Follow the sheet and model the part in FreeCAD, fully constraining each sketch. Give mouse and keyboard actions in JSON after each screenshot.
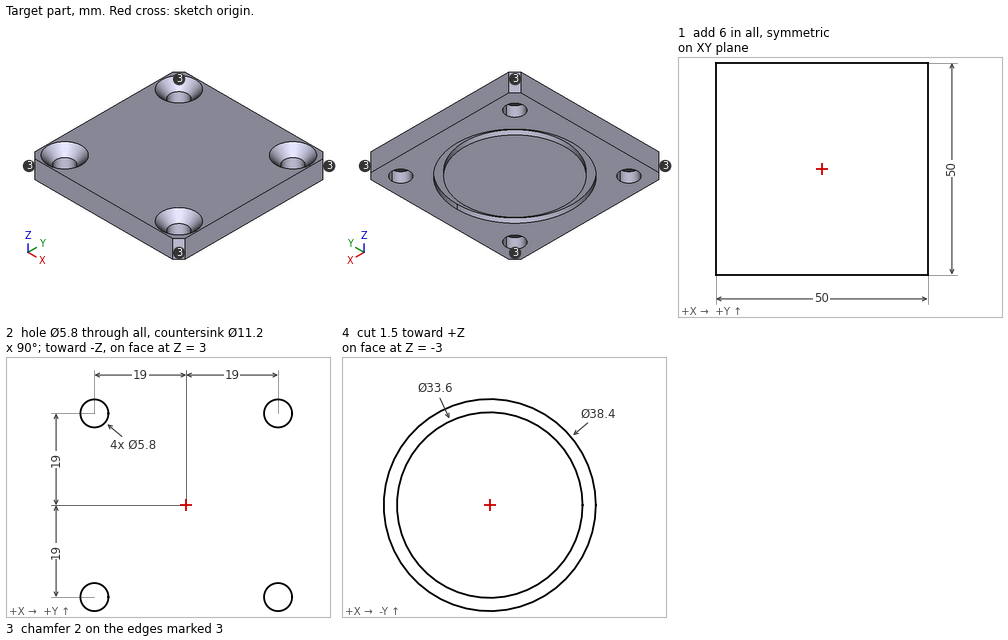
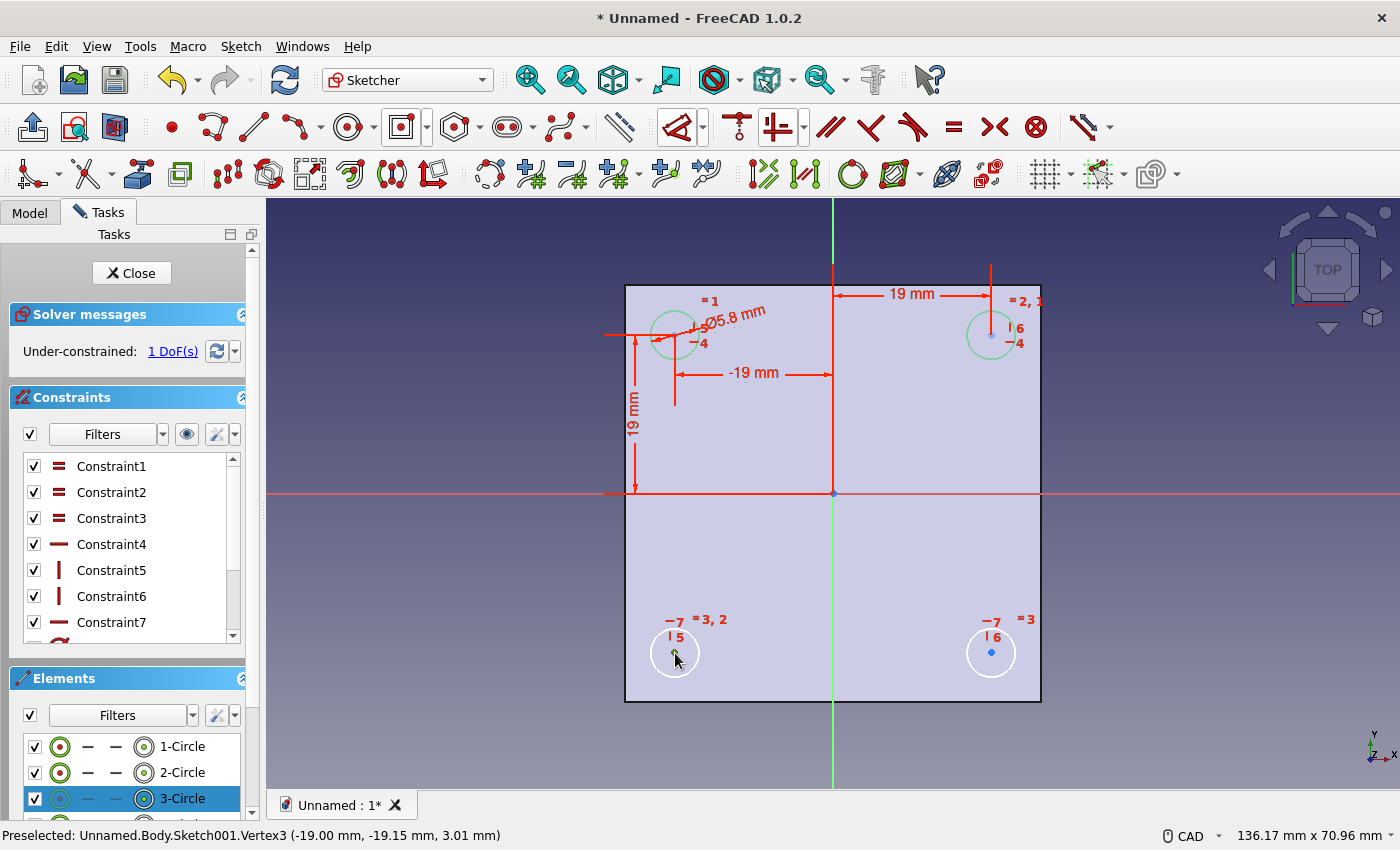
{"action": "key", "text": "i"}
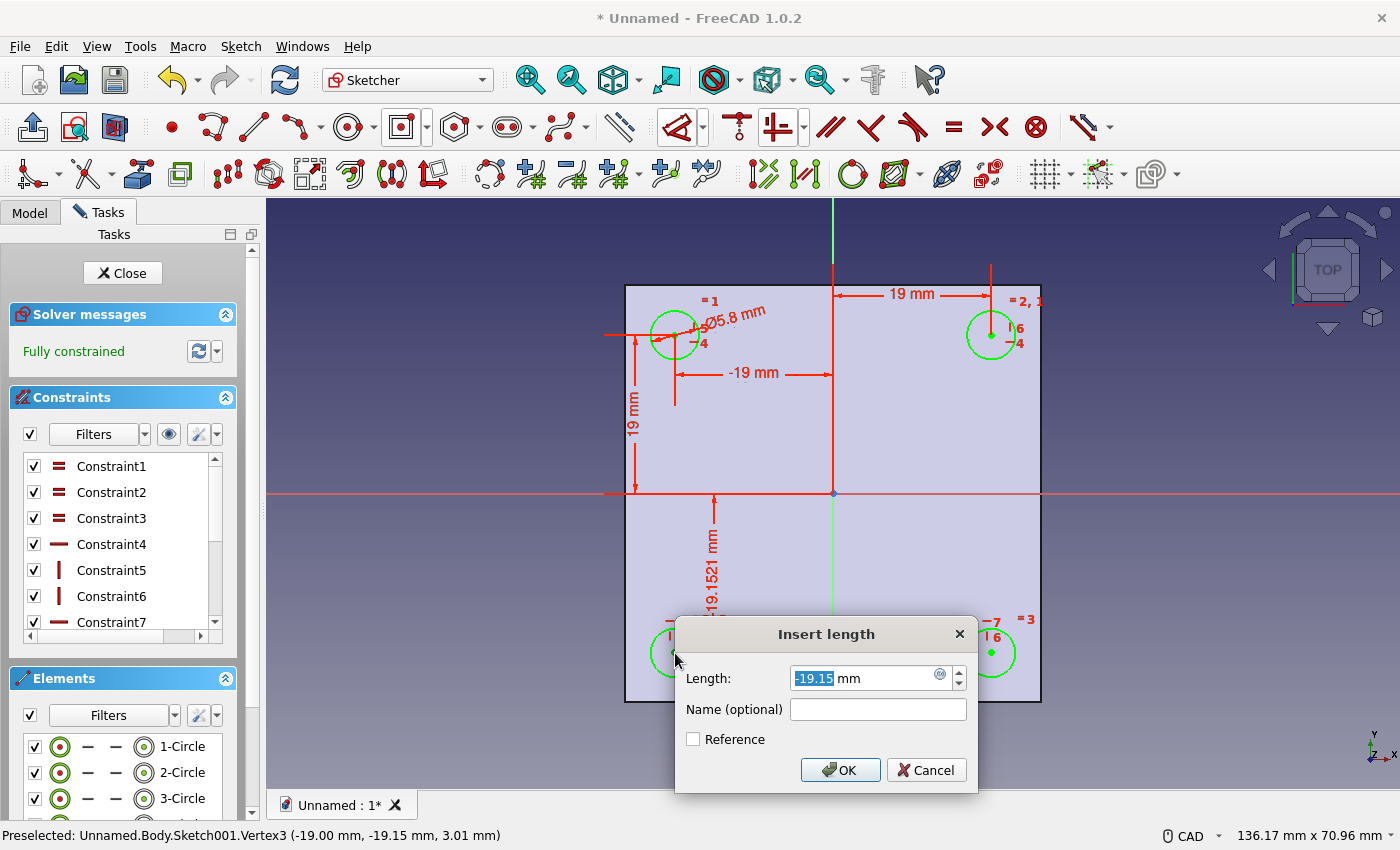
{"action": "type", "text": "-19"}
{"action": "key", "text": "Return"}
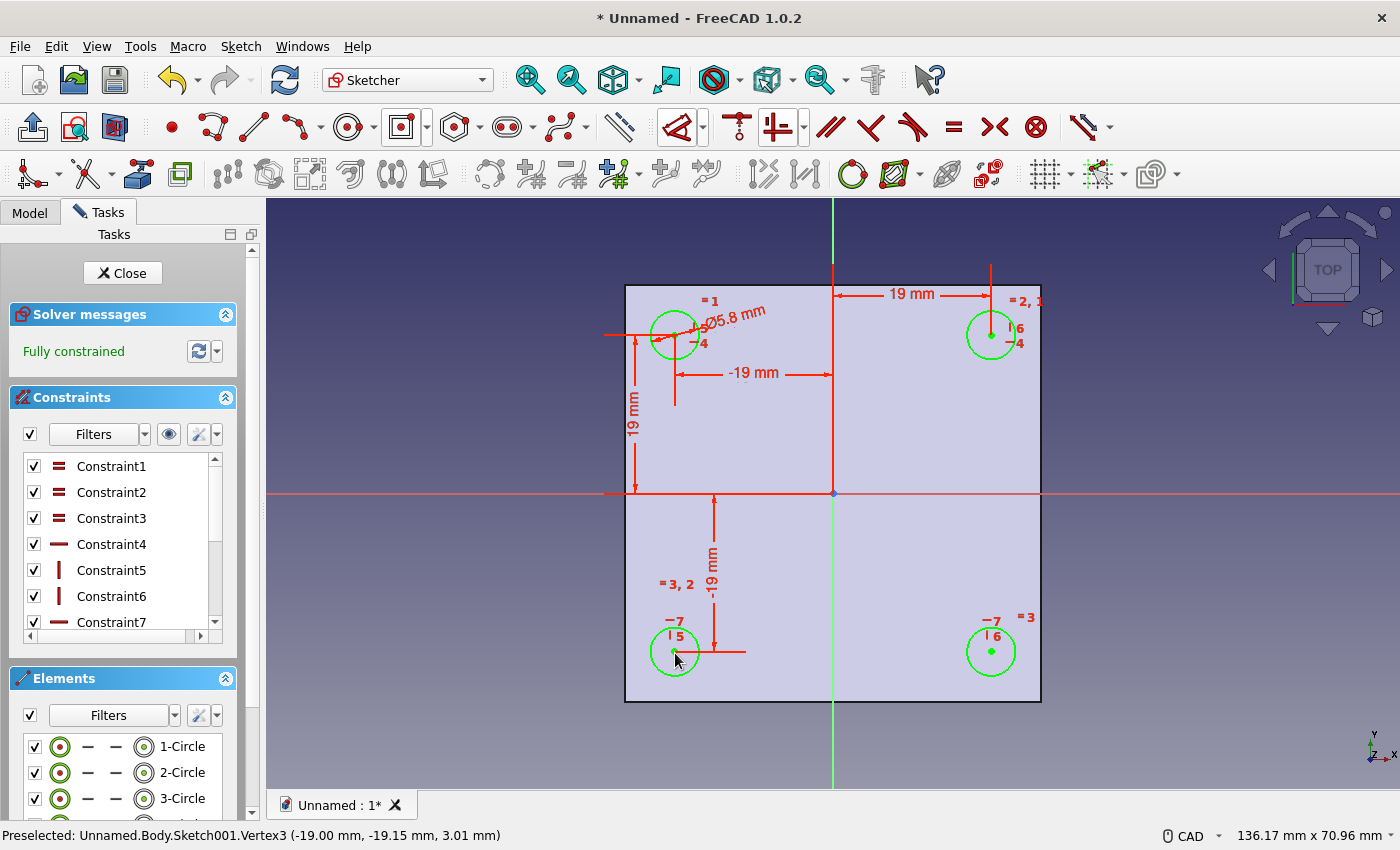
{"action": "left_click", "coordinate": [123, 273]}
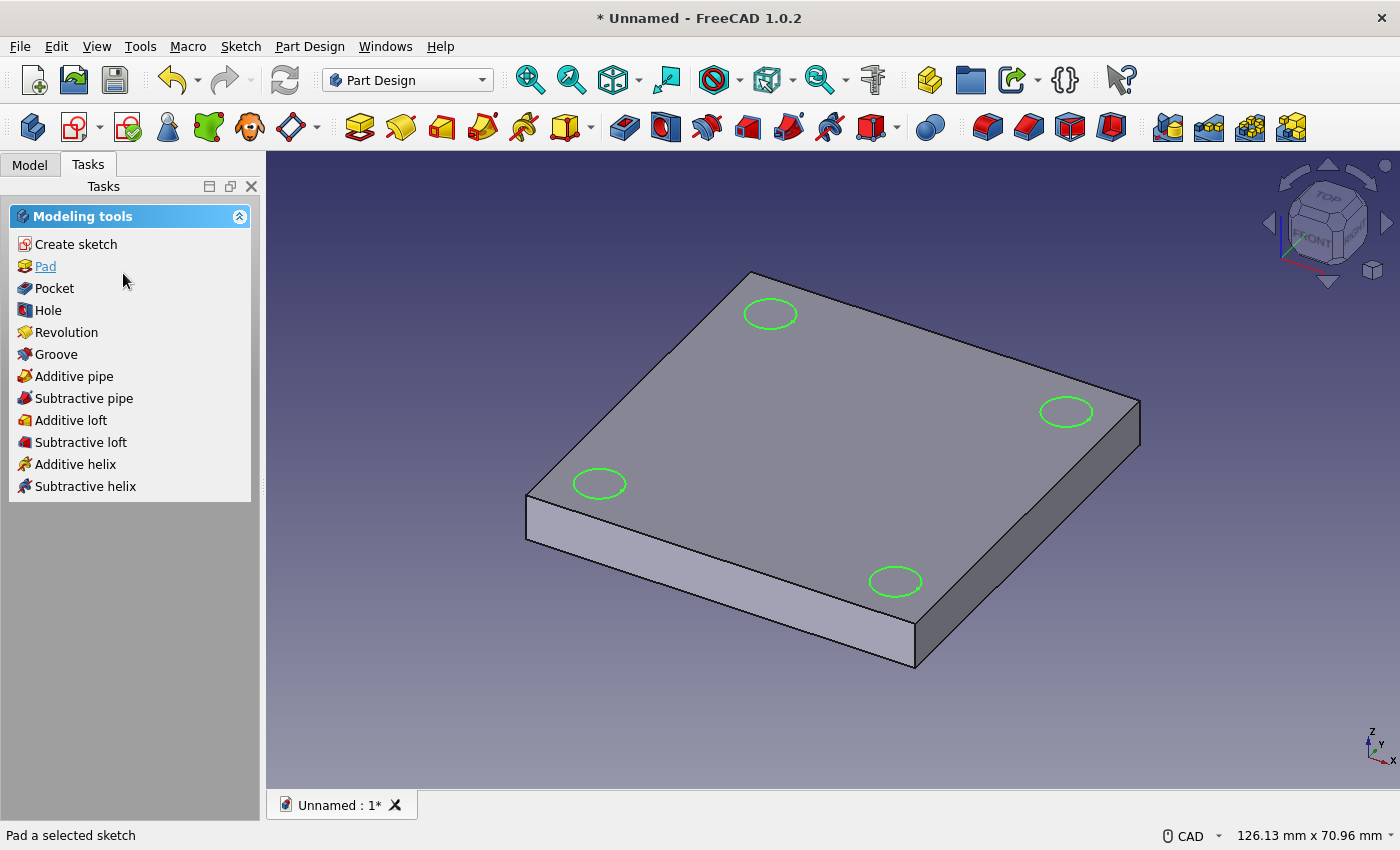
{"action": "left_click", "coordinate": [666, 128]}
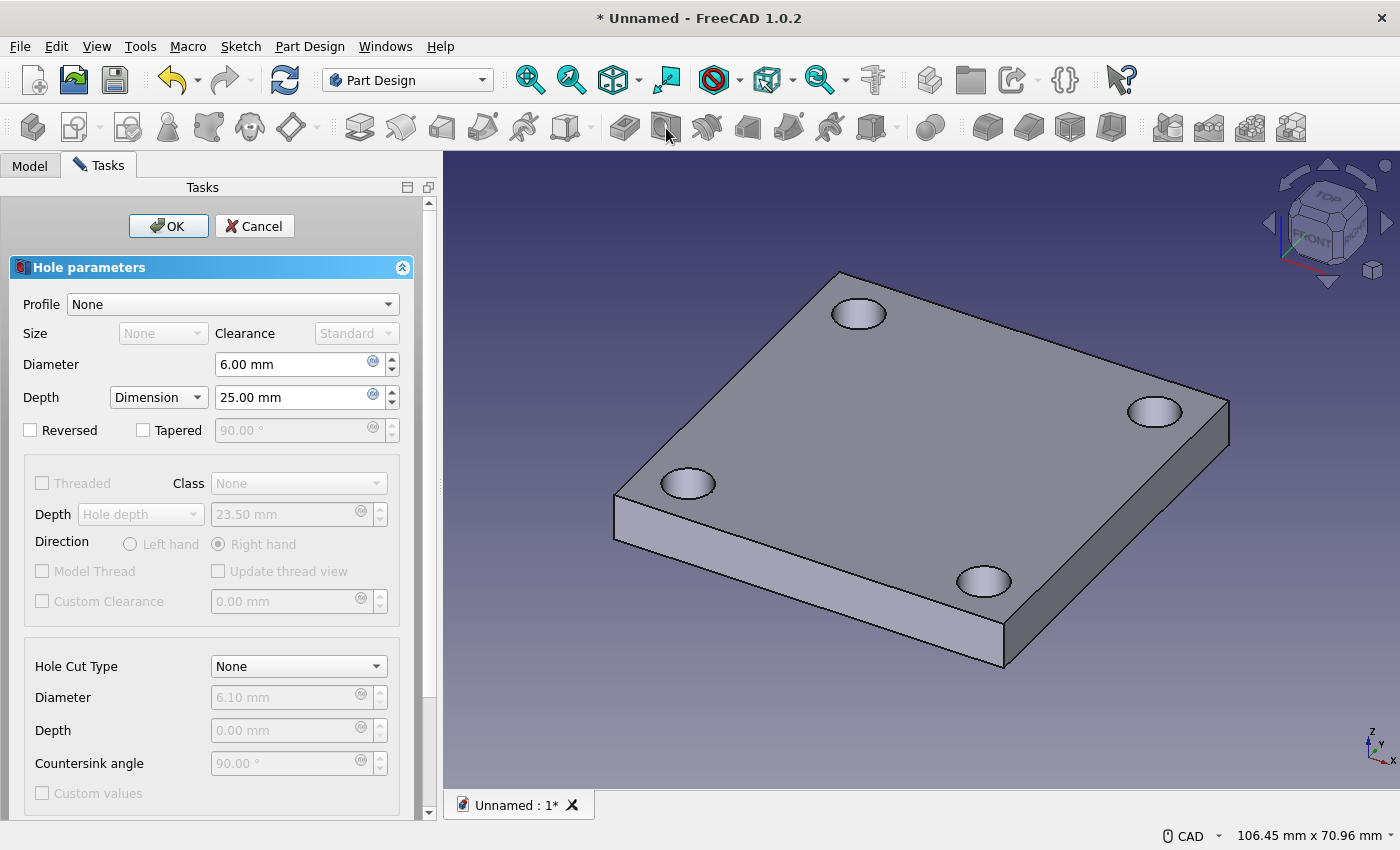
{"action": "triple_click", "coordinate": [300, 364]}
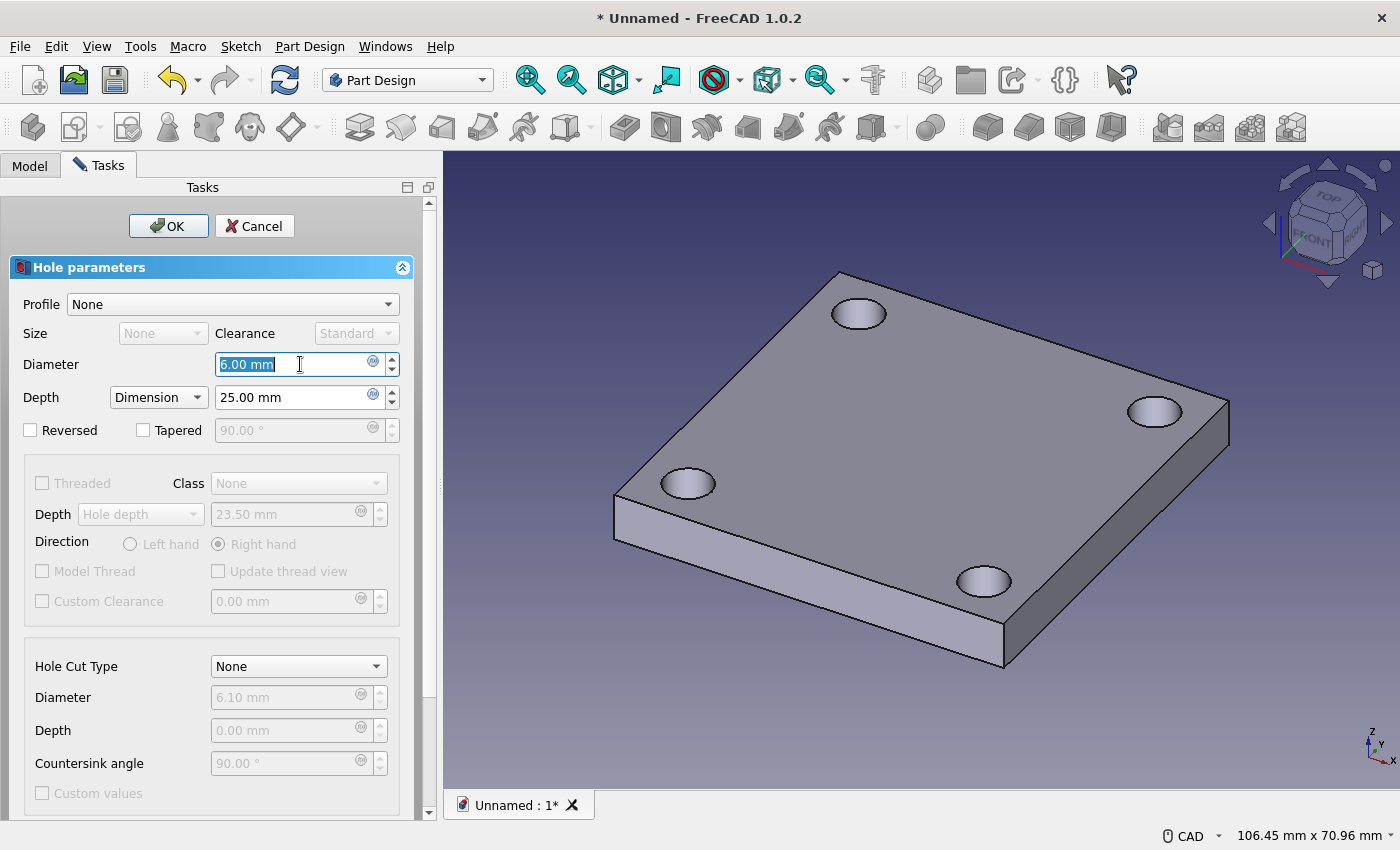
{"action": "type", "text": "5.8"}
{"action": "key", "text": "Tab"}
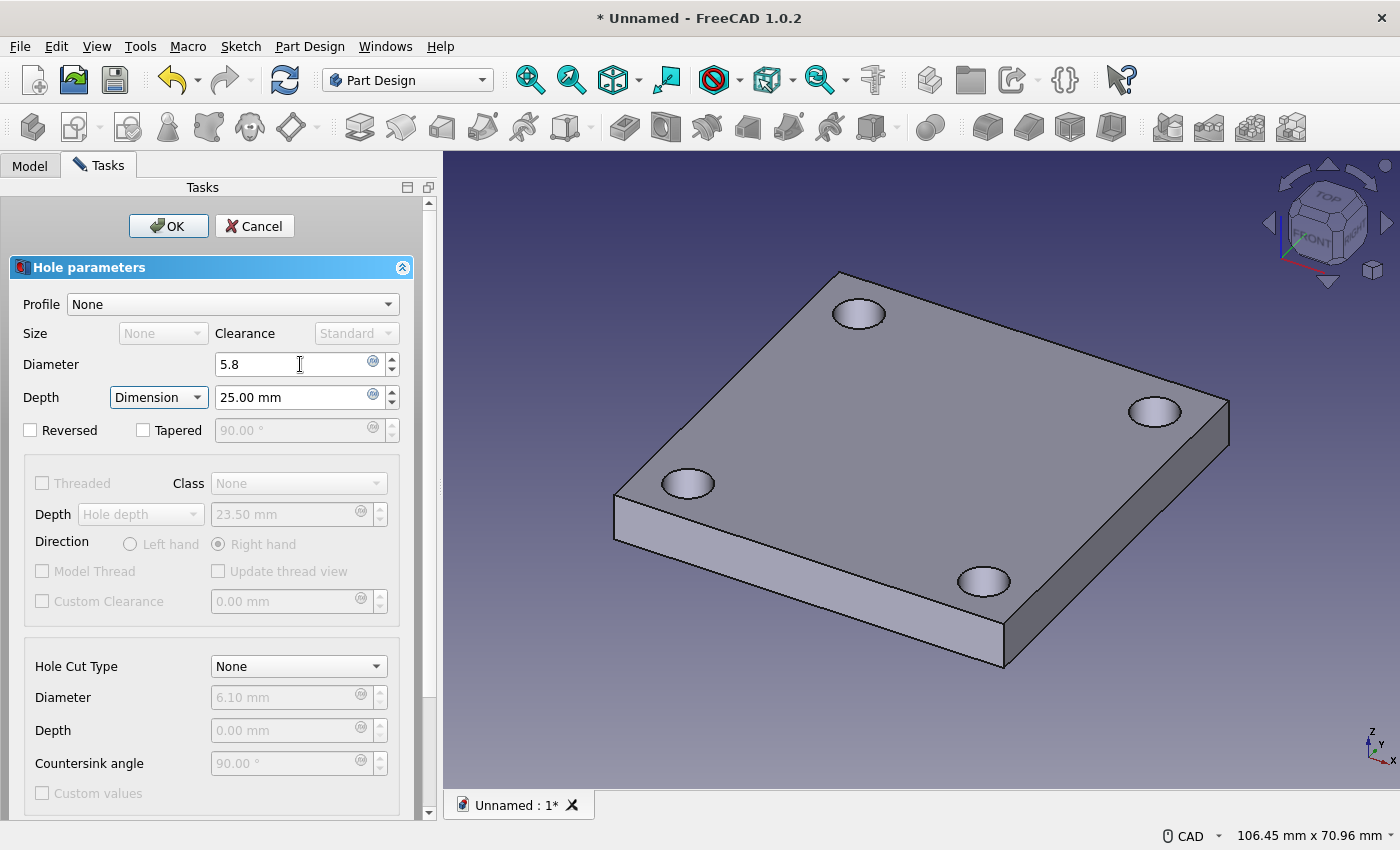
{"action": "left_click", "coordinate": [160, 398]}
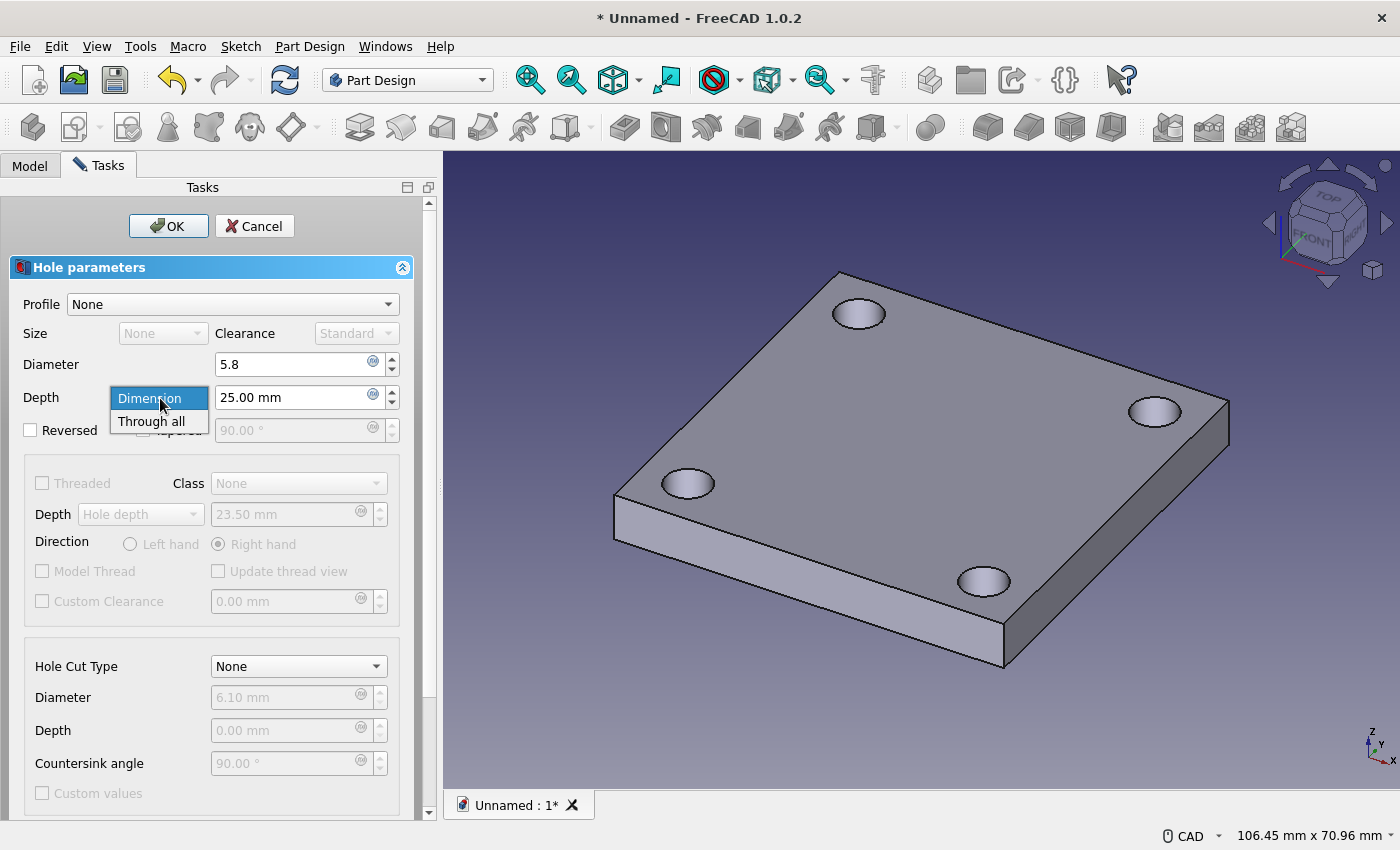
{"action": "left_click", "coordinate": [158, 422]}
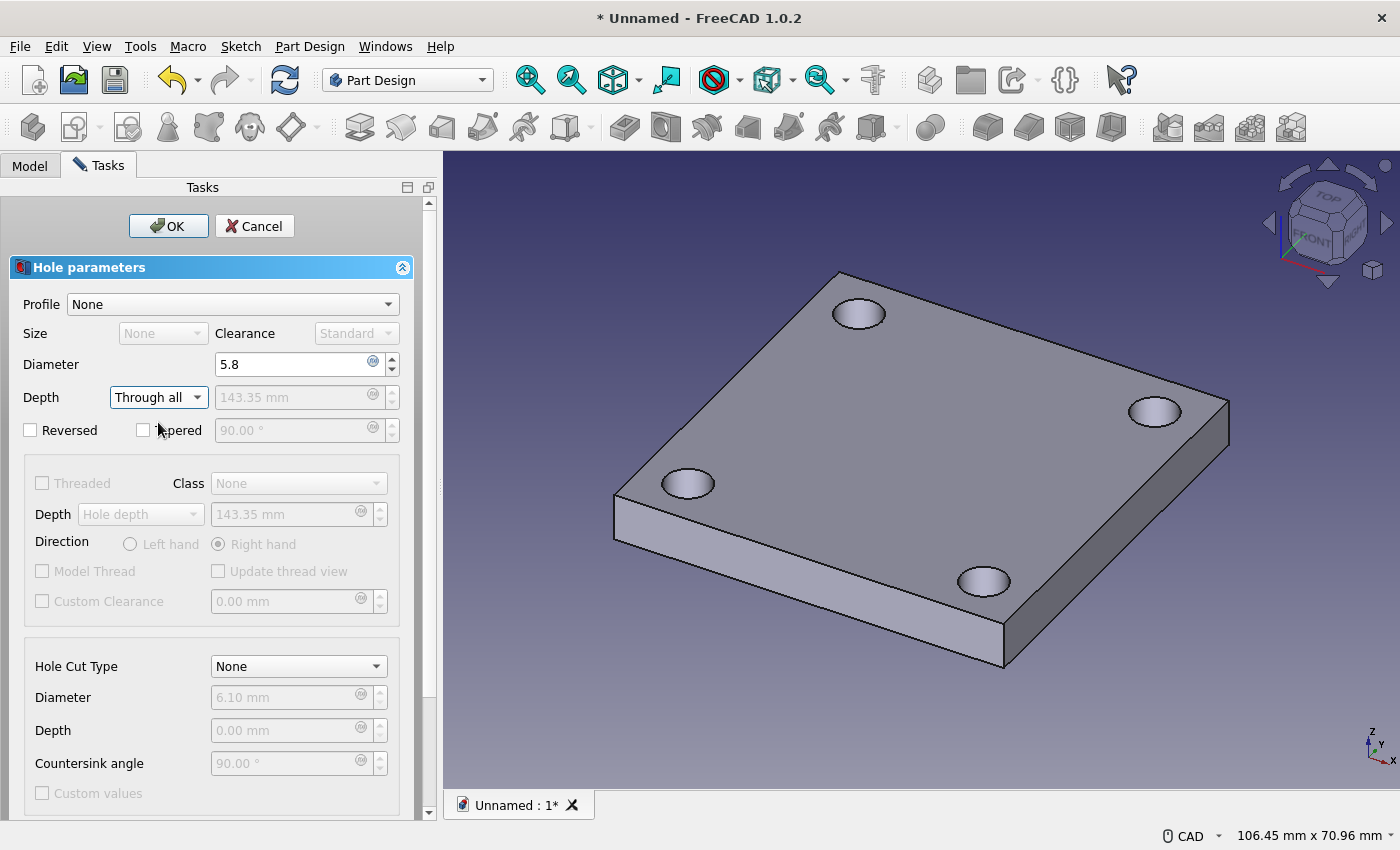
{"action": "left_click", "coordinate": [300, 666]}